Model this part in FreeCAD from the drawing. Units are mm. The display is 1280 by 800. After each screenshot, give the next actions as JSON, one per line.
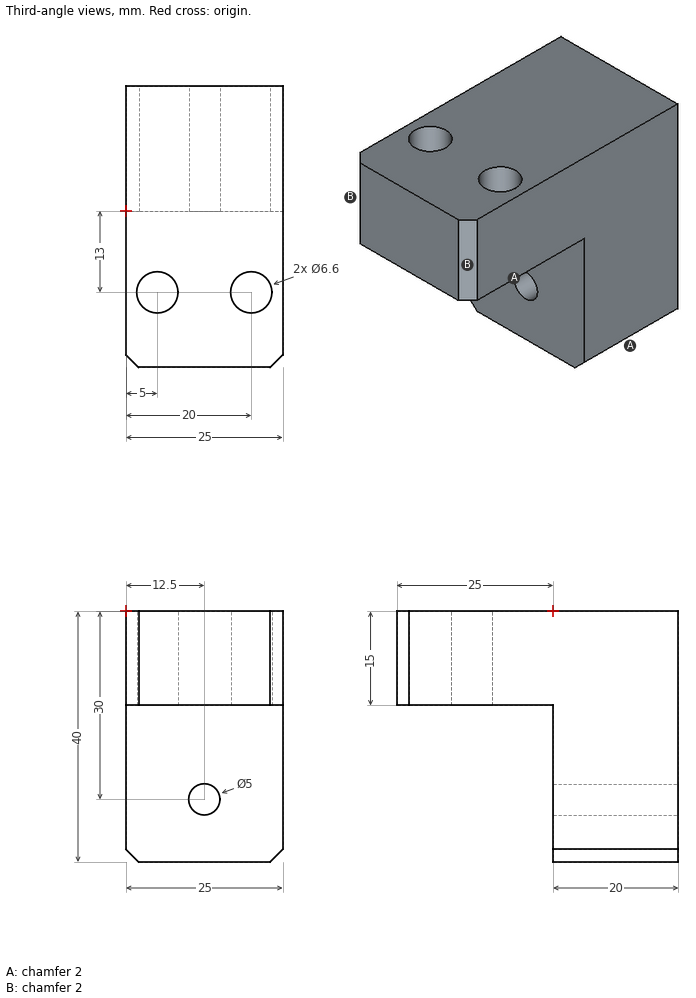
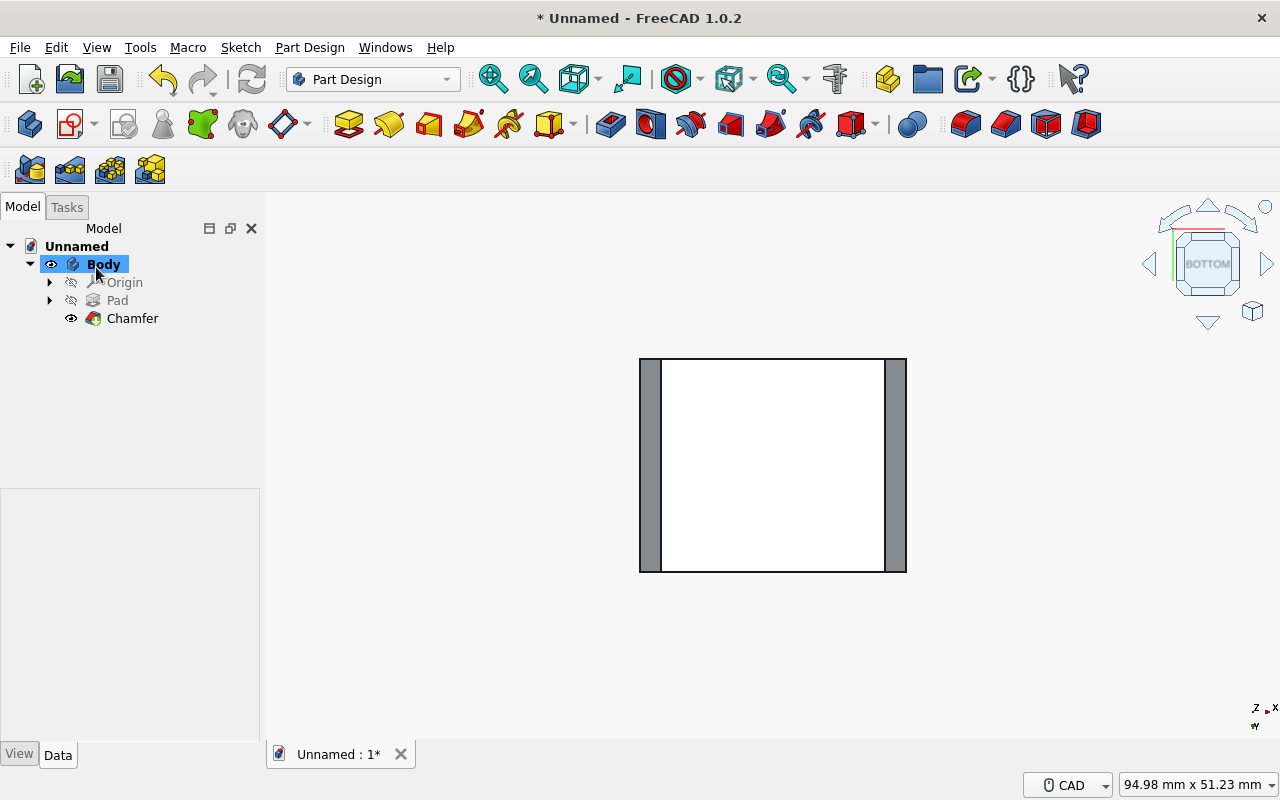
{"action": "left_click", "coordinate": [494, 80]}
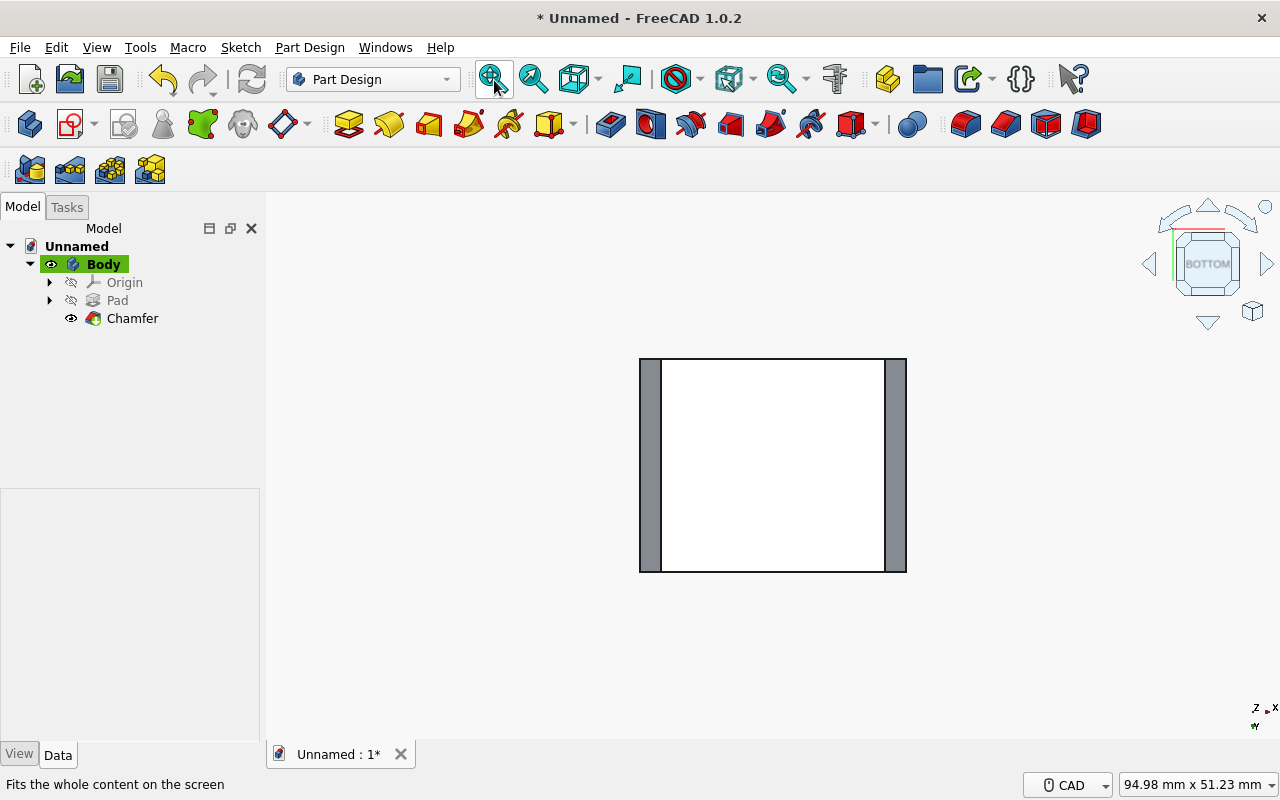
{"action": "key", "text": "0"}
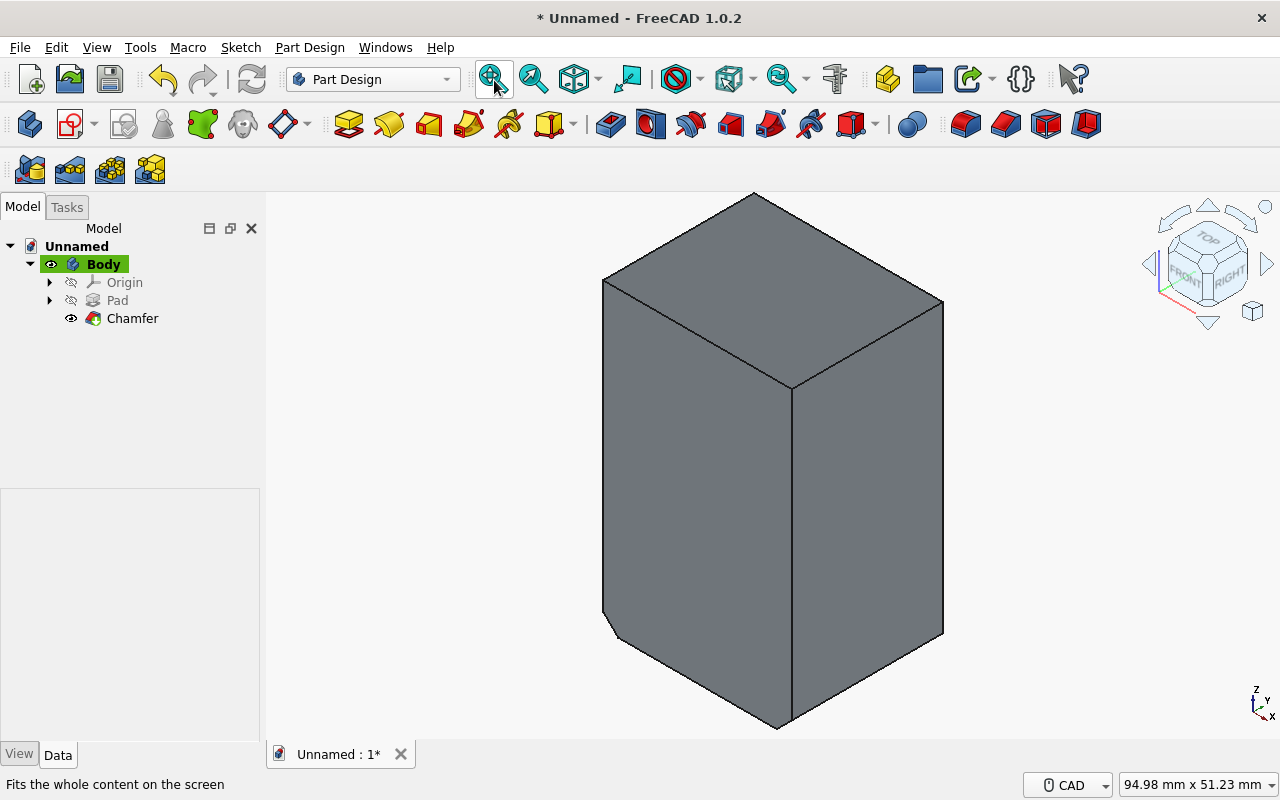
{"action": "left_click", "coordinate": [698, 458]}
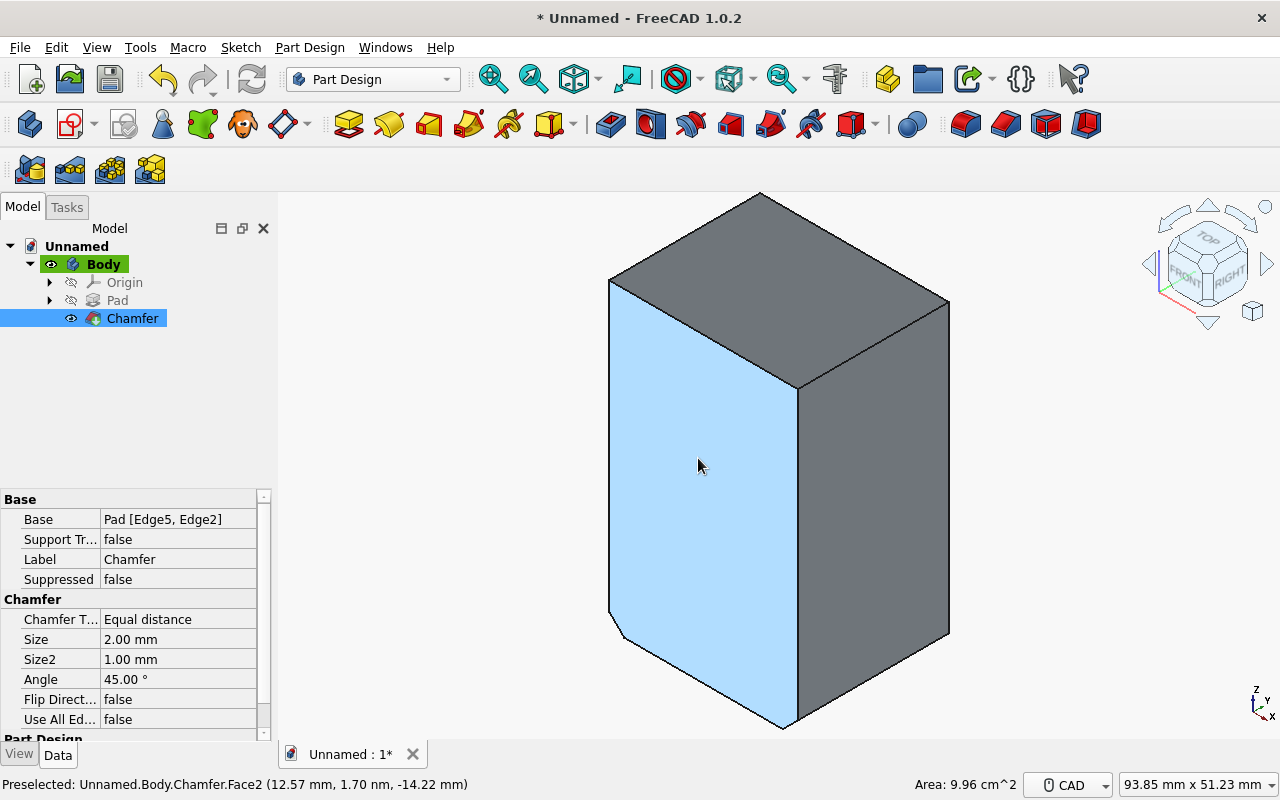
{"action": "left_click", "coordinate": [70, 124]}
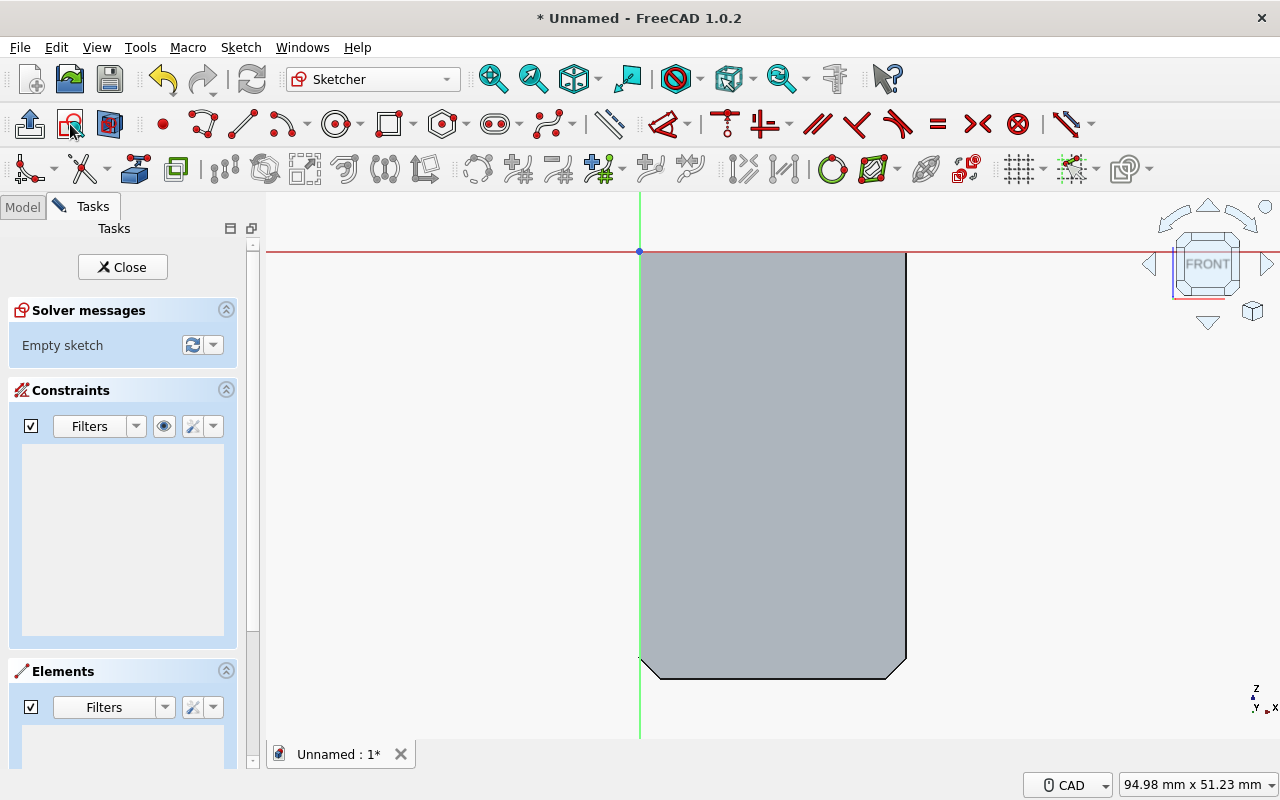
{"action": "scroll", "coordinate": [787, 593], "scroll_direction": "up", "scroll_amount": 9}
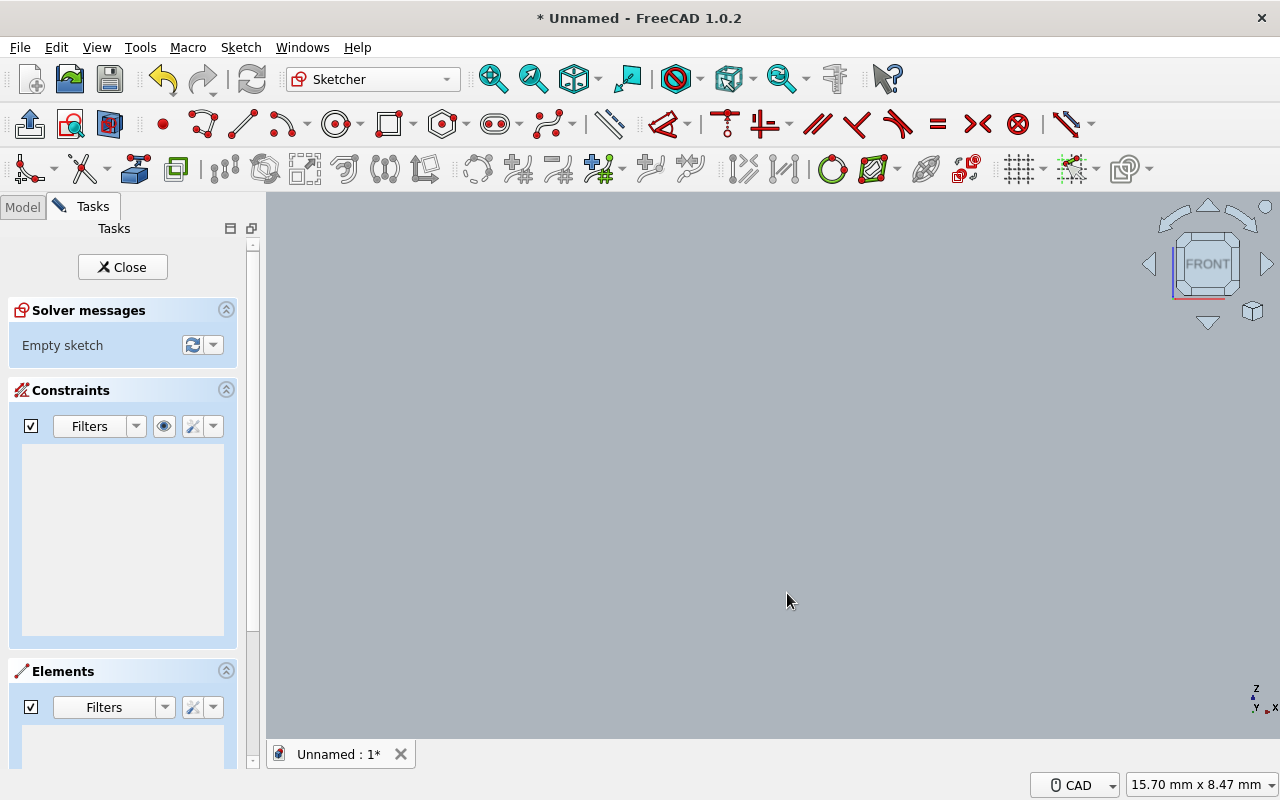
{"action": "key", "text": "g c"}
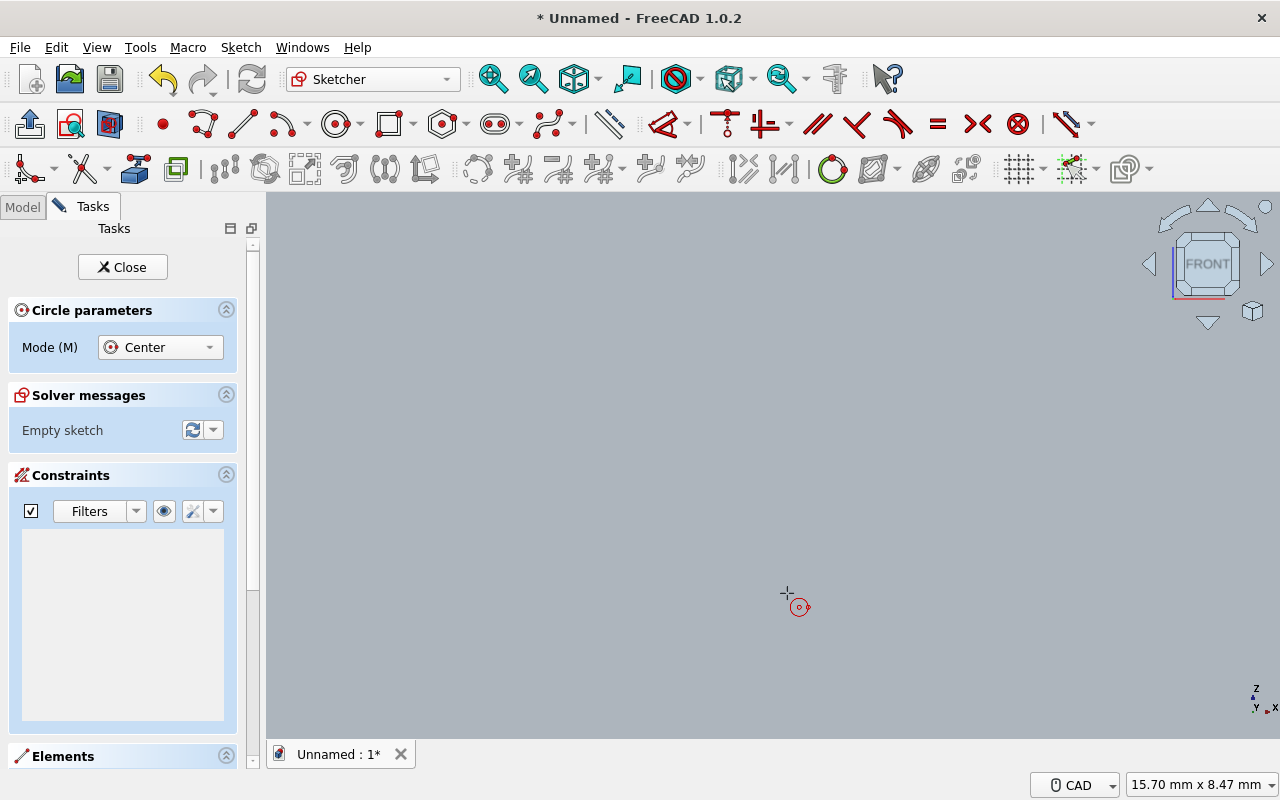
{"action": "left_click", "coordinate": [700, 464]}
{"action": "left_click", "coordinate": [814, 350]}
{"action": "key", "text": "Escape"}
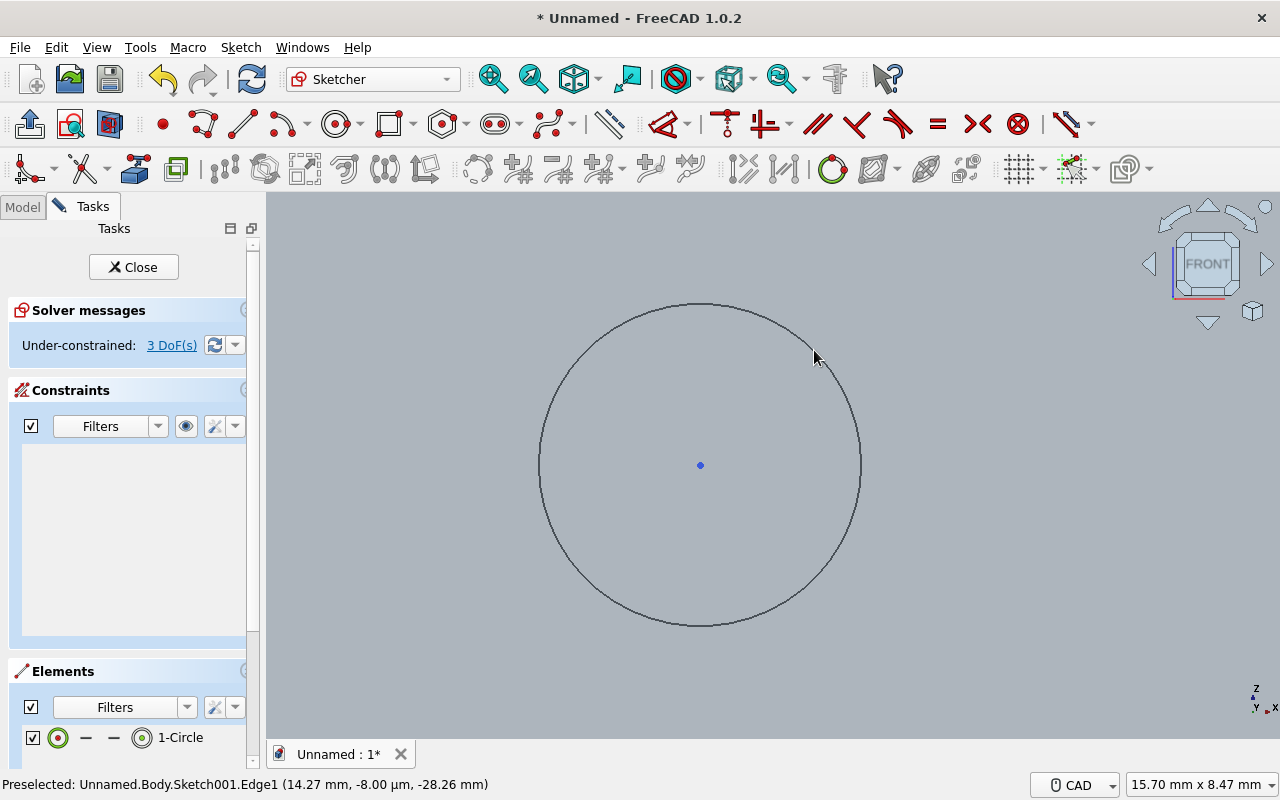
{"action": "left_click", "coordinate": [814, 351]}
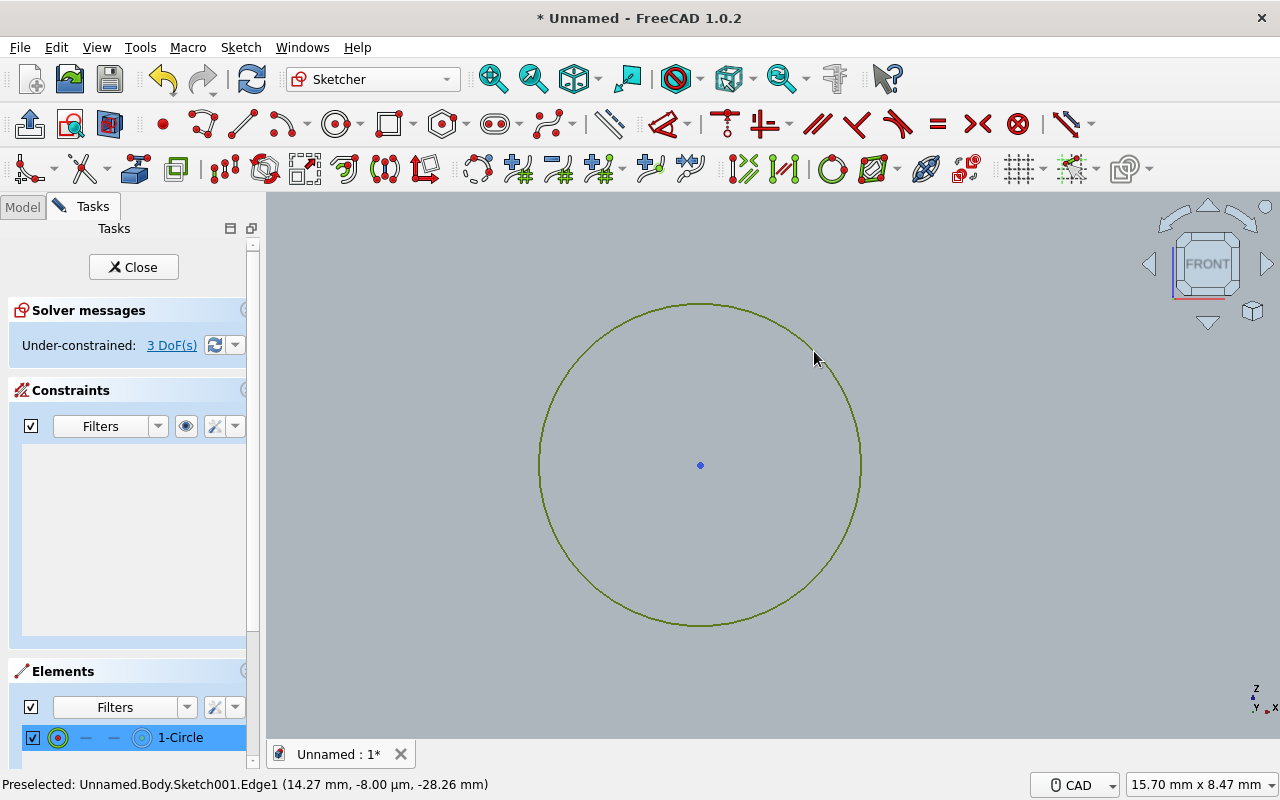
{"action": "key", "text": "k o"}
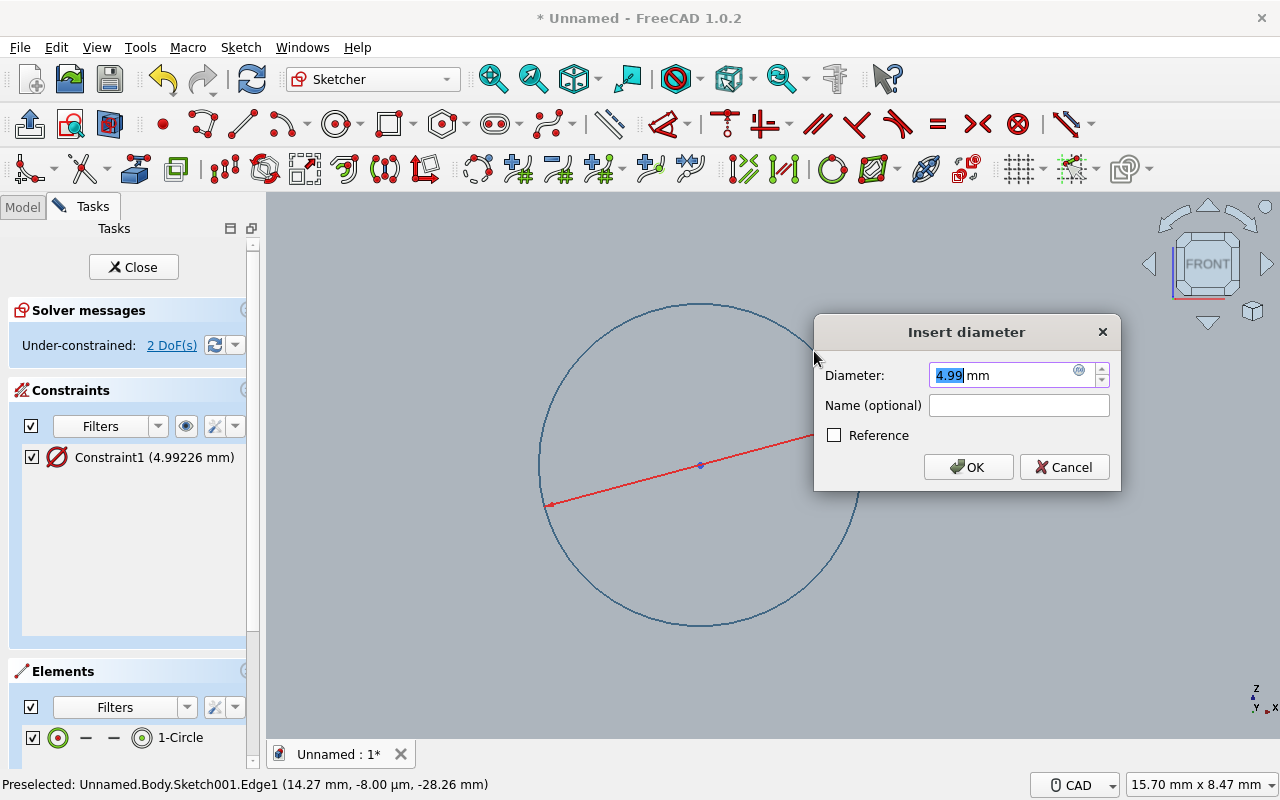
{"action": "type", "text": "5"}
{"action": "key", "text": "Return"}